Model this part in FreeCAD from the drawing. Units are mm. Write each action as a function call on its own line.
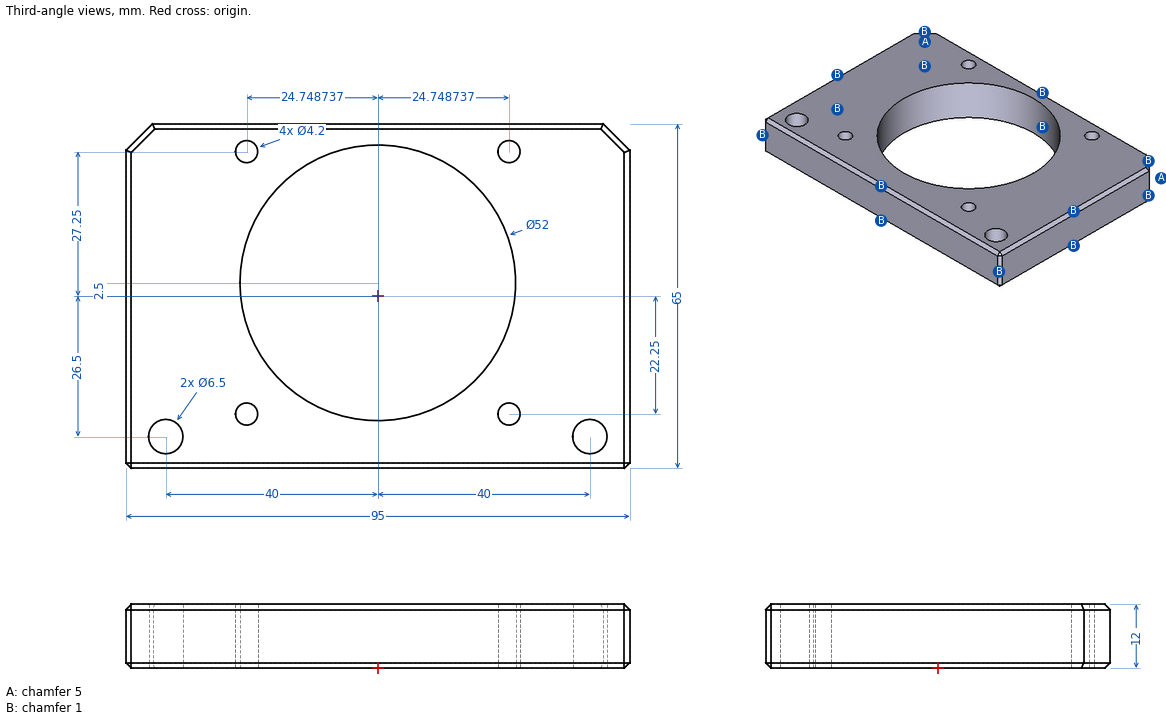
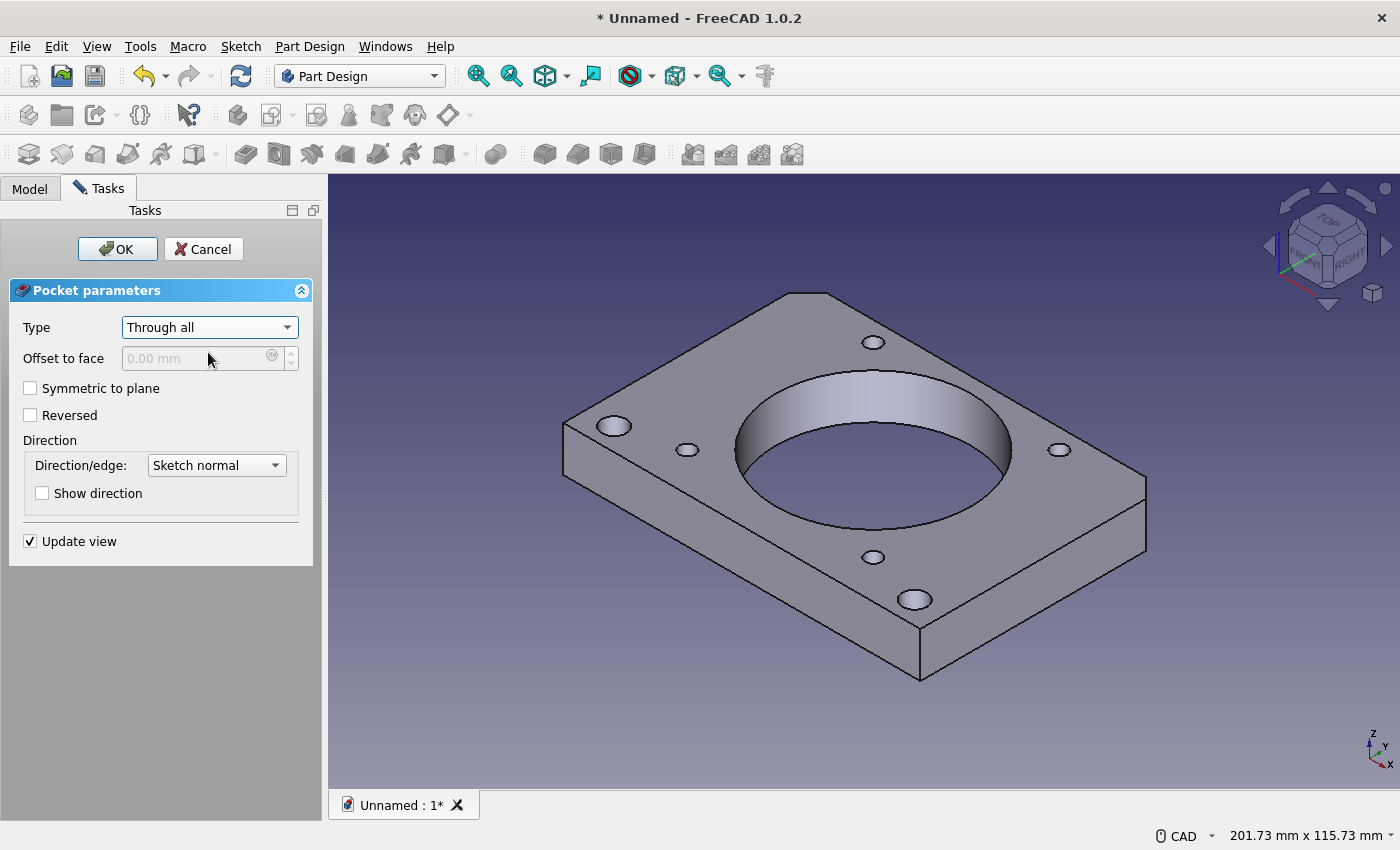
click(118, 249)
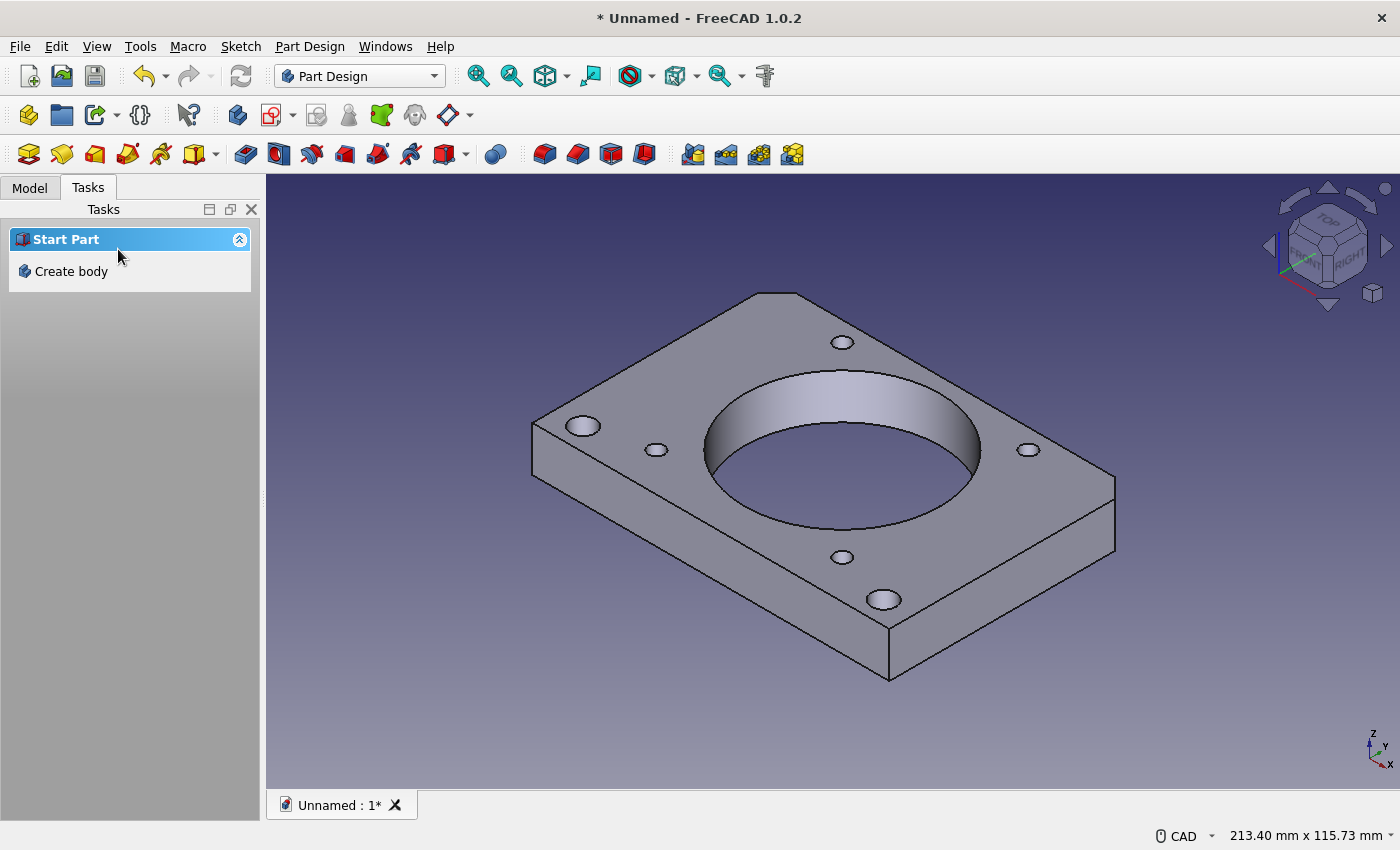
click(864, 639)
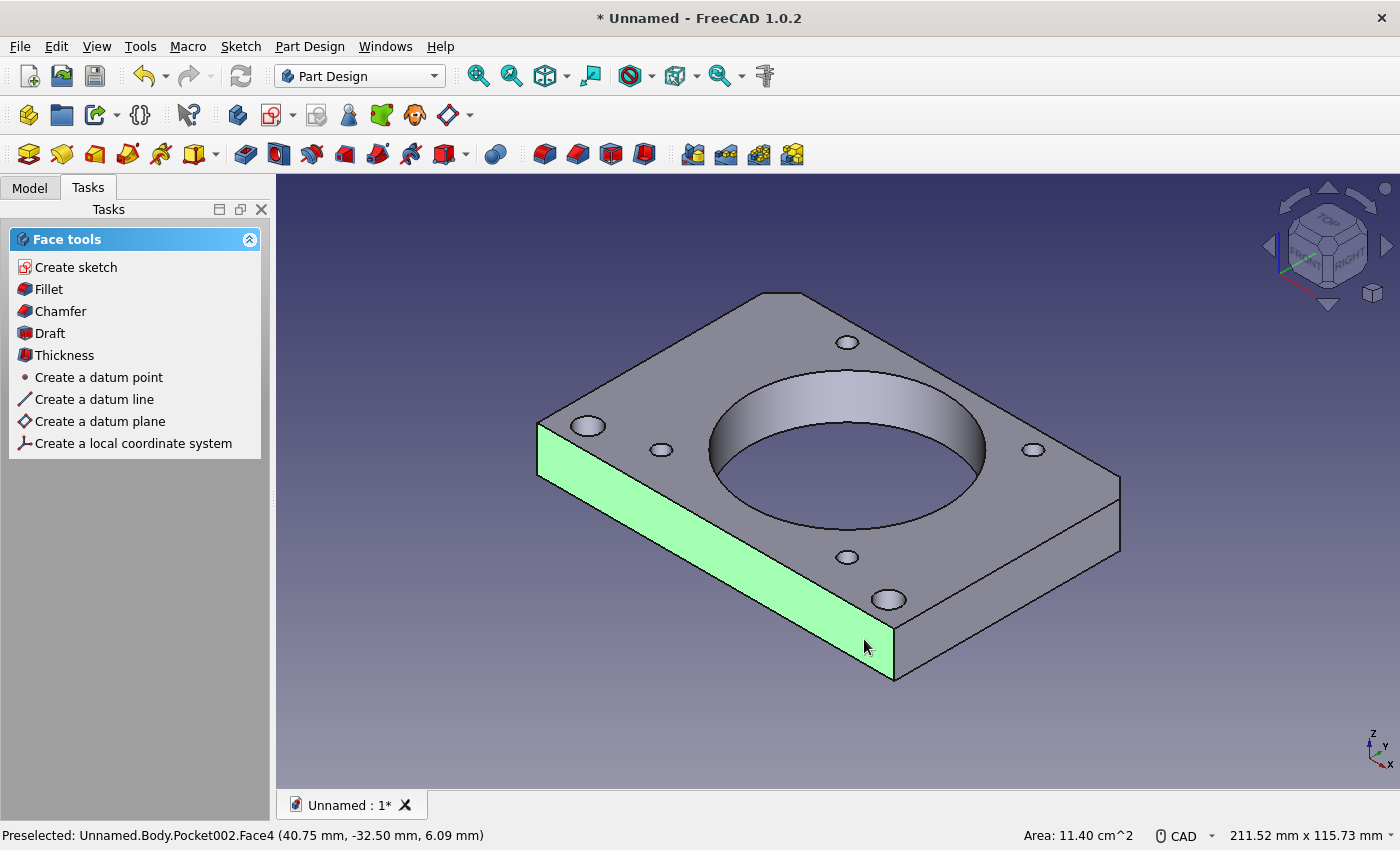
click(1007, 563, ctrl)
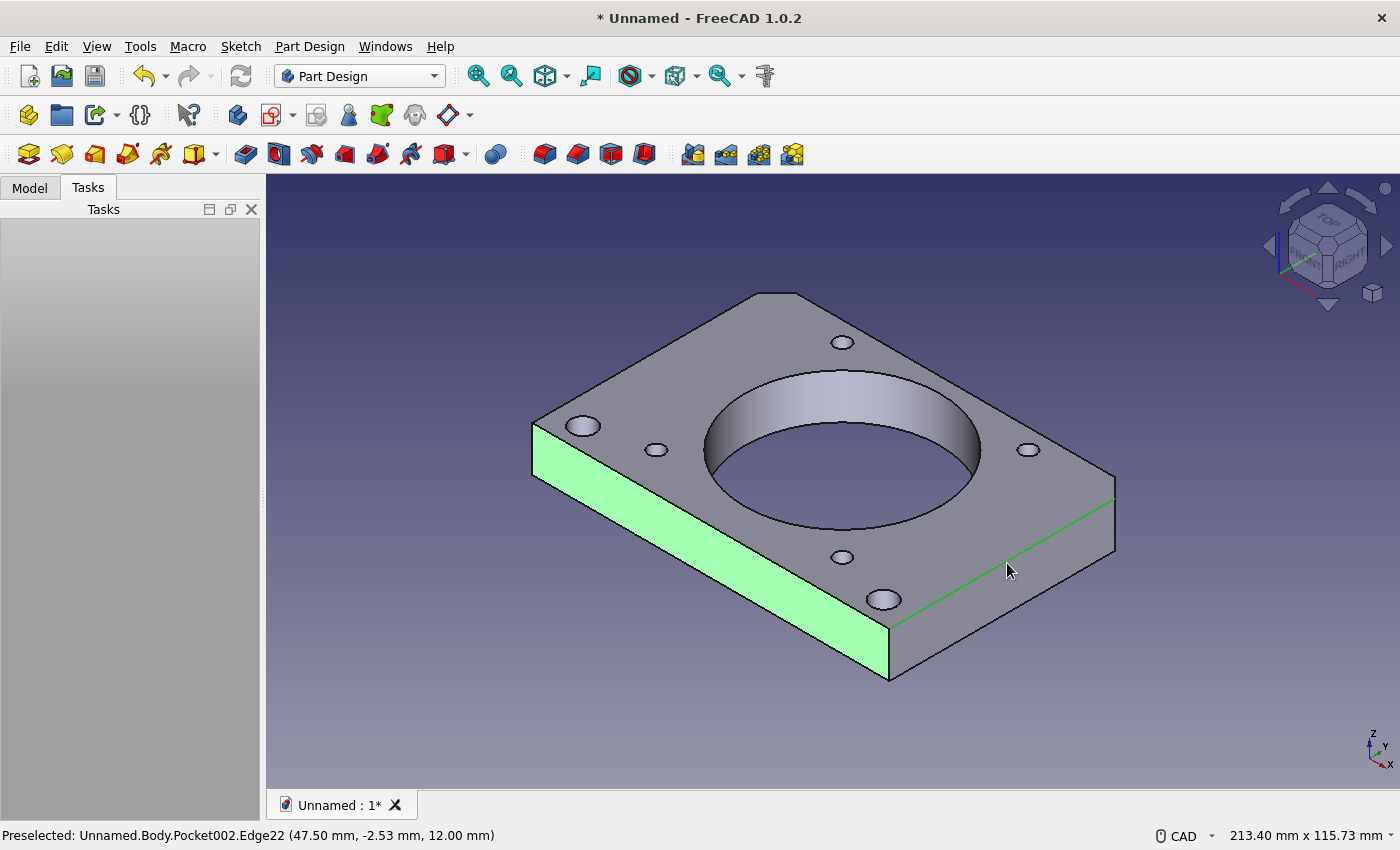
click(1115, 489, ctrl)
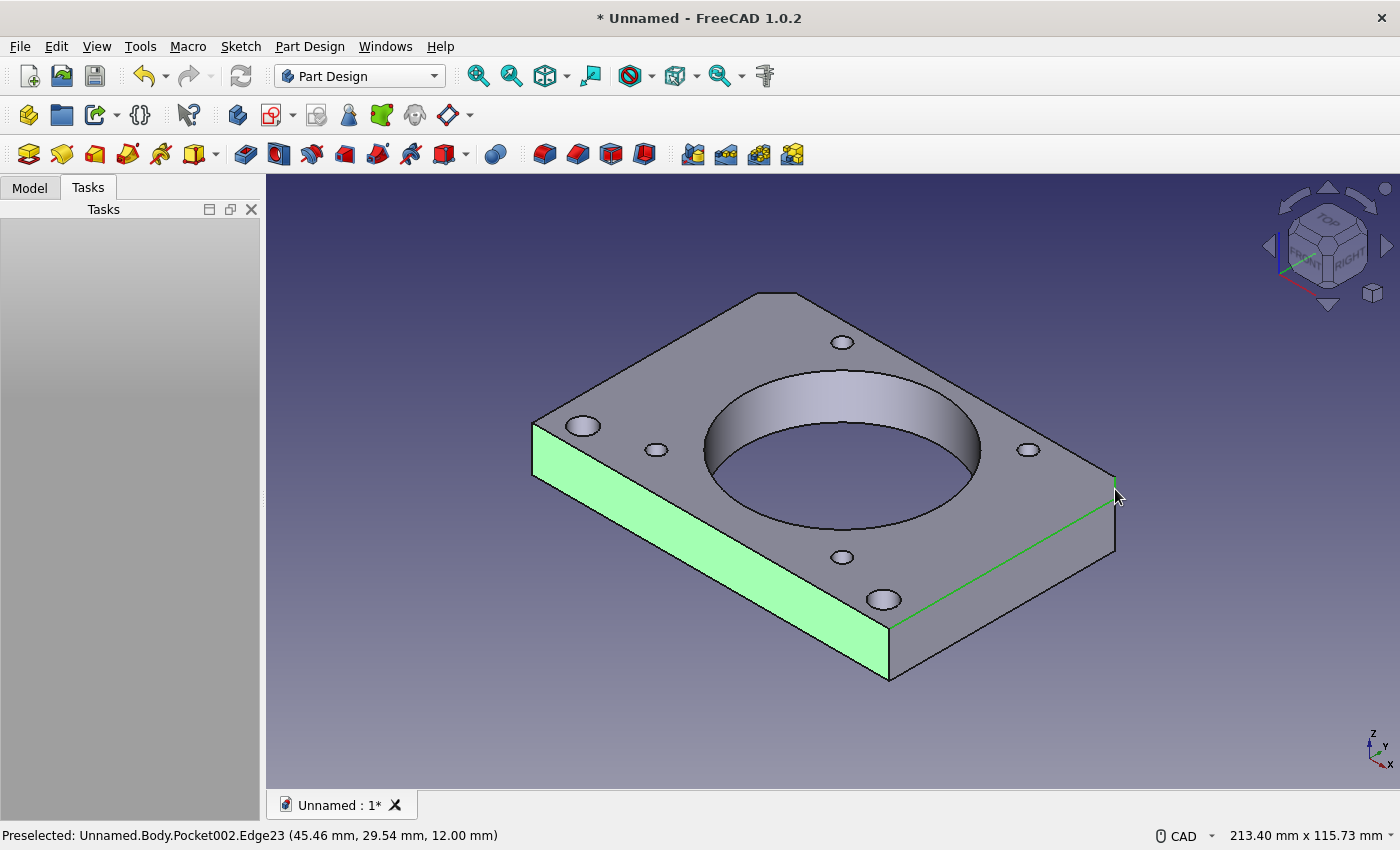
key(2)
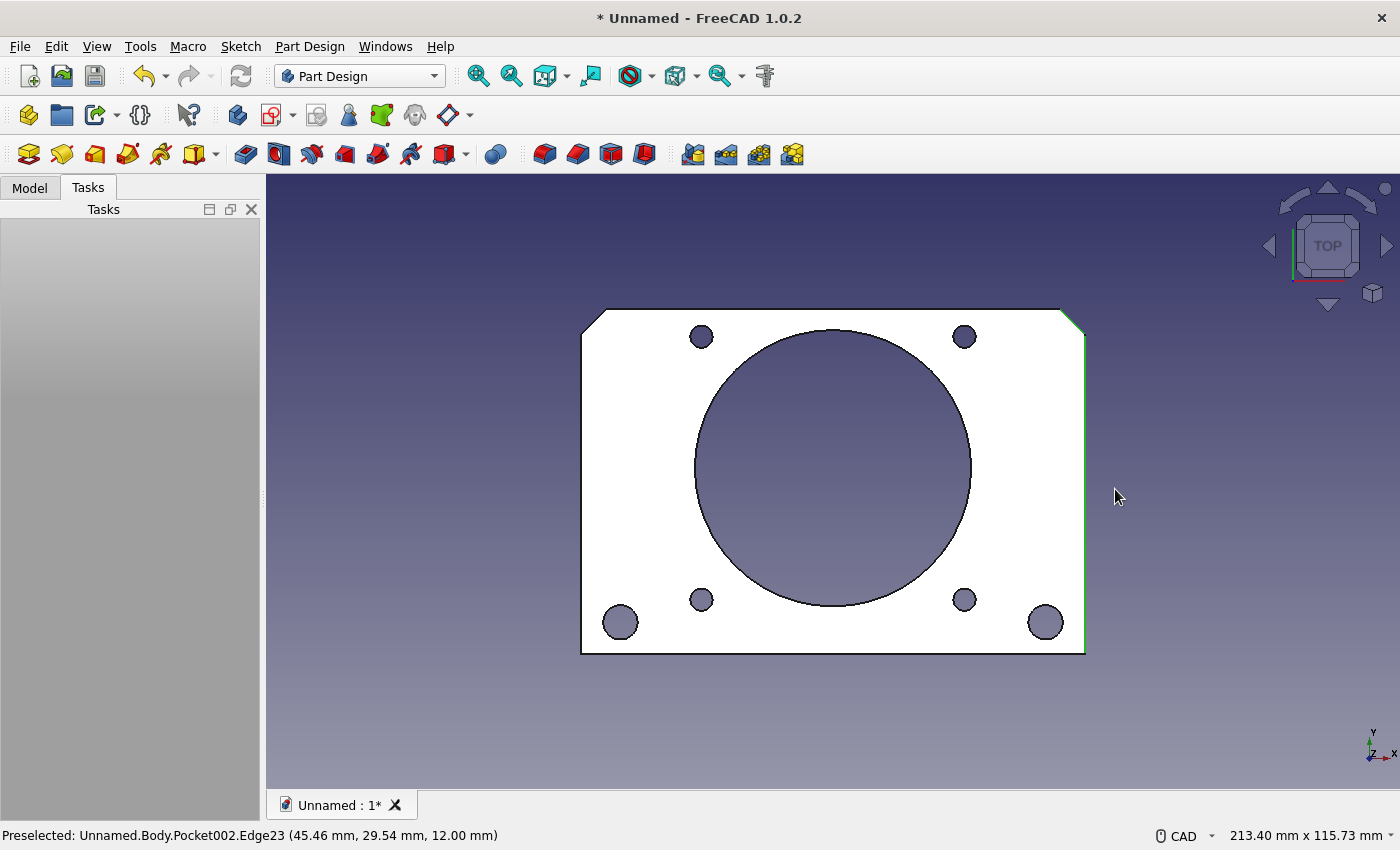
click(833, 308, ctrl)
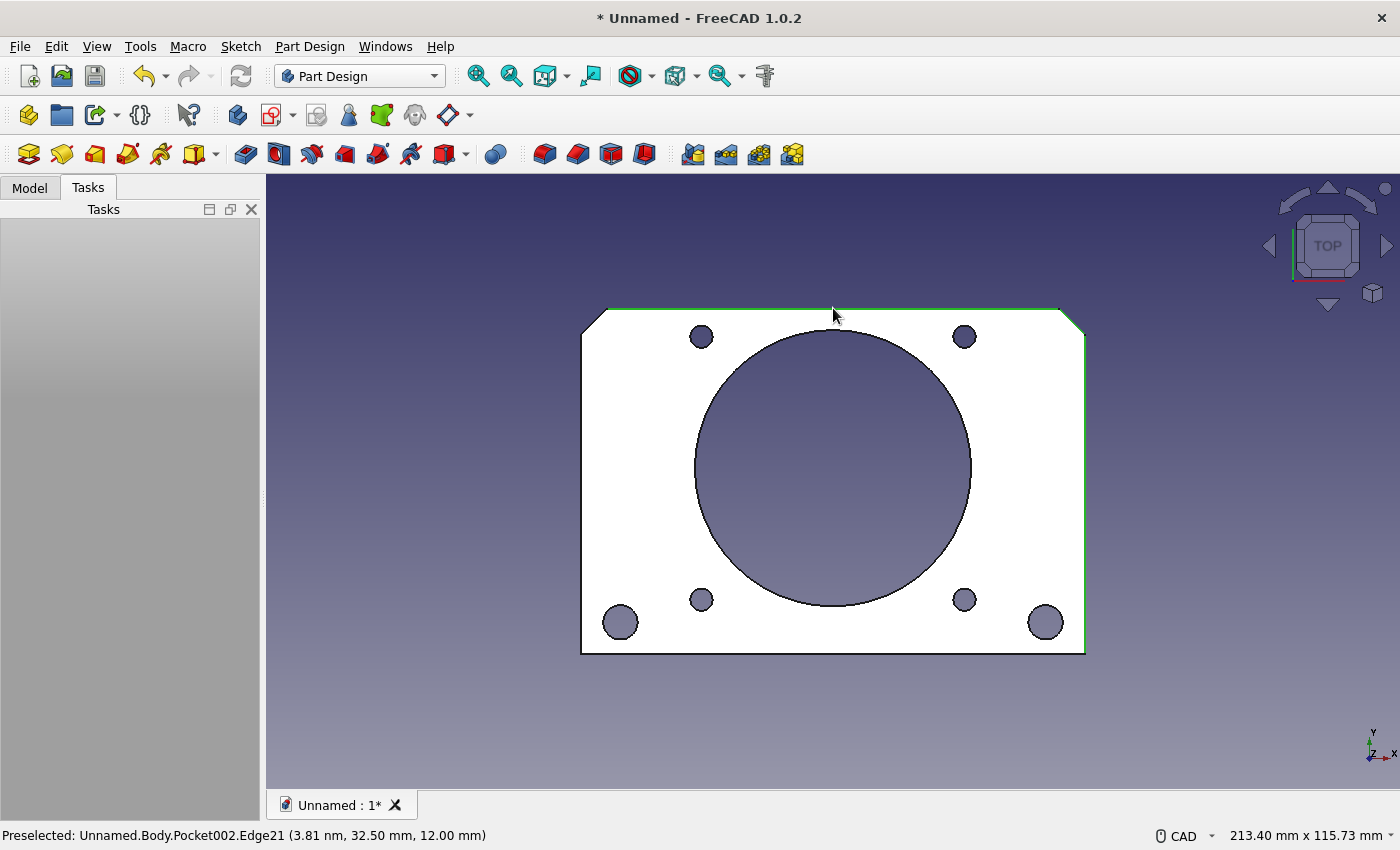
click(581, 494, ctrl)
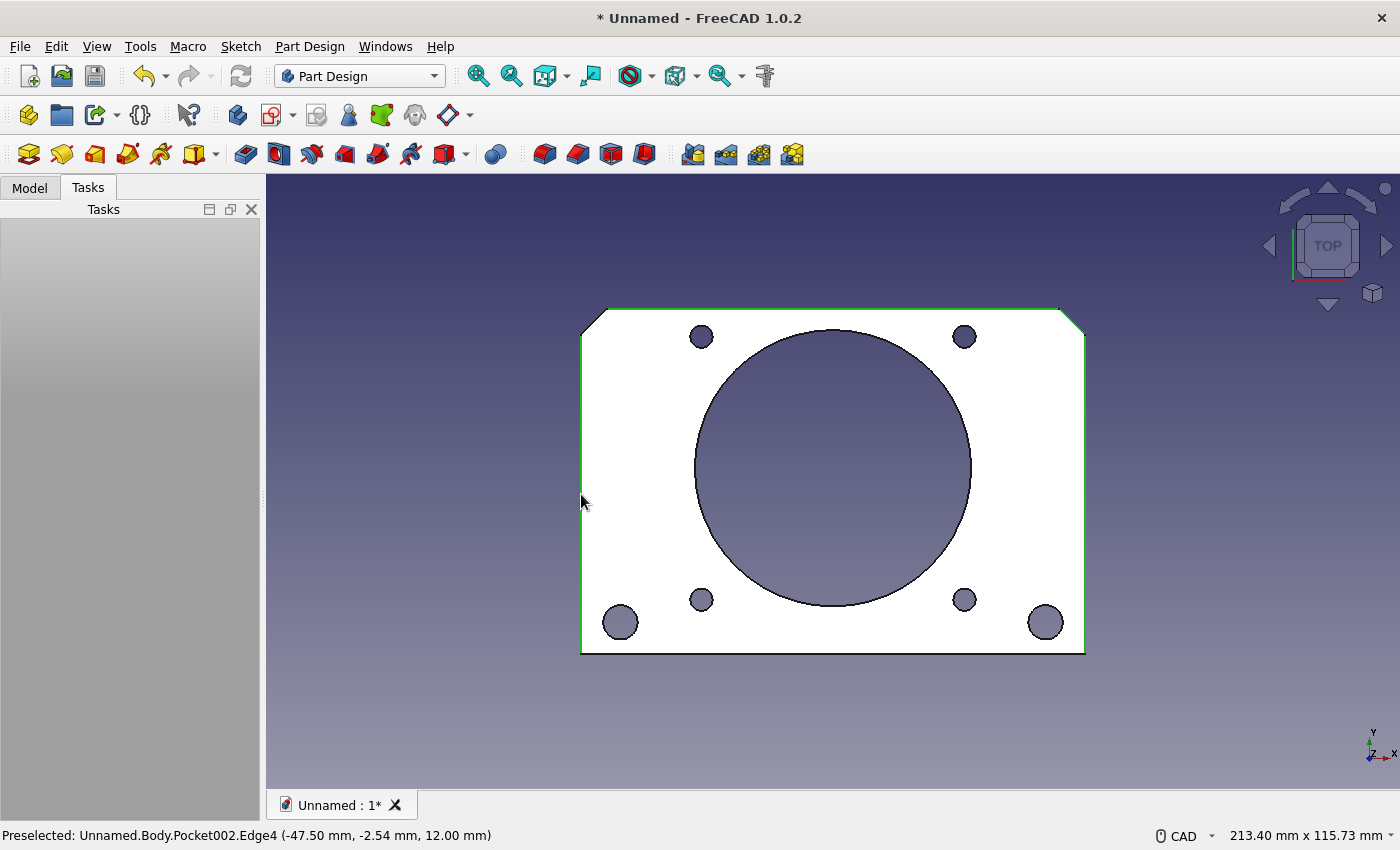
click(594, 321, ctrl)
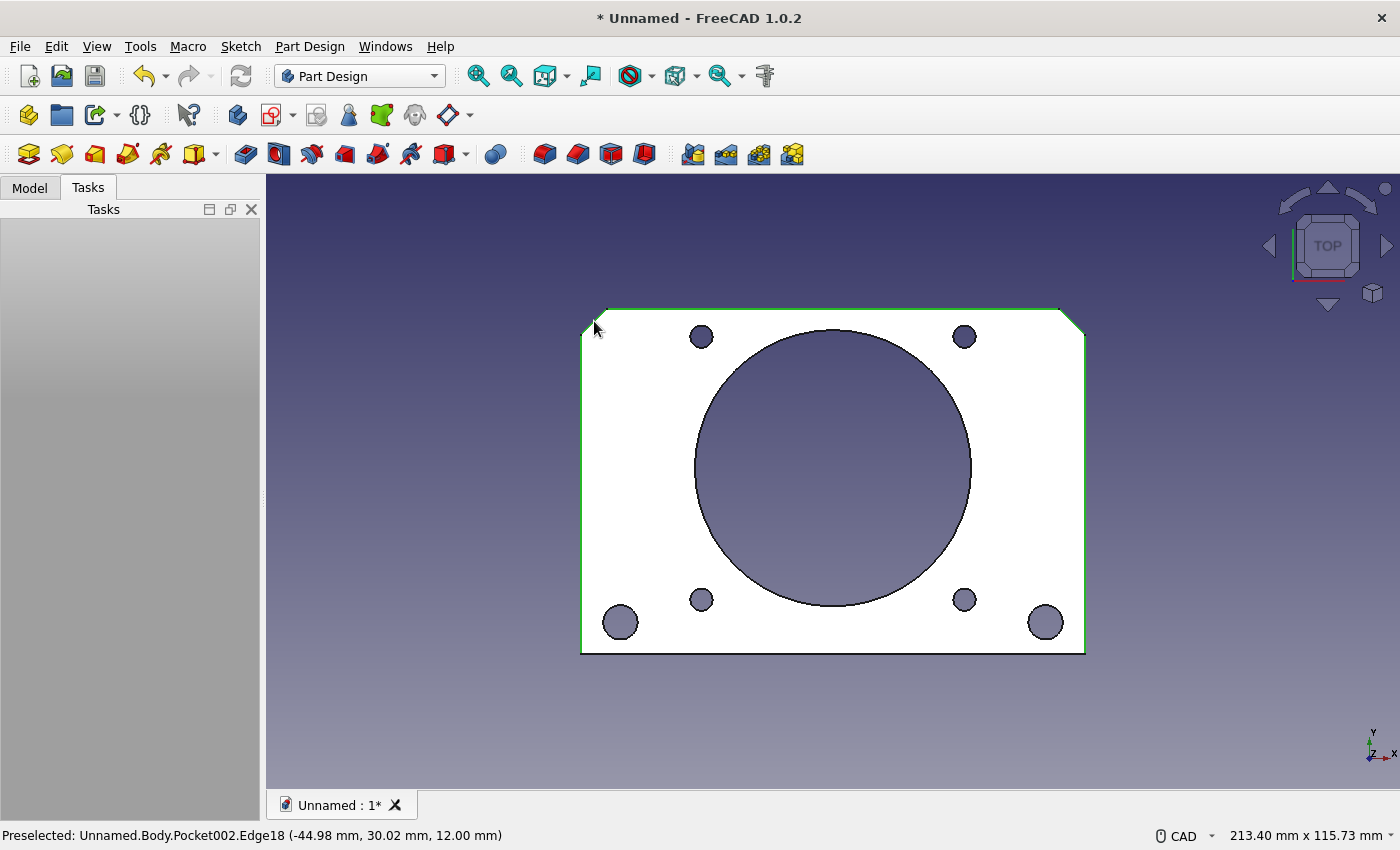
key(0)